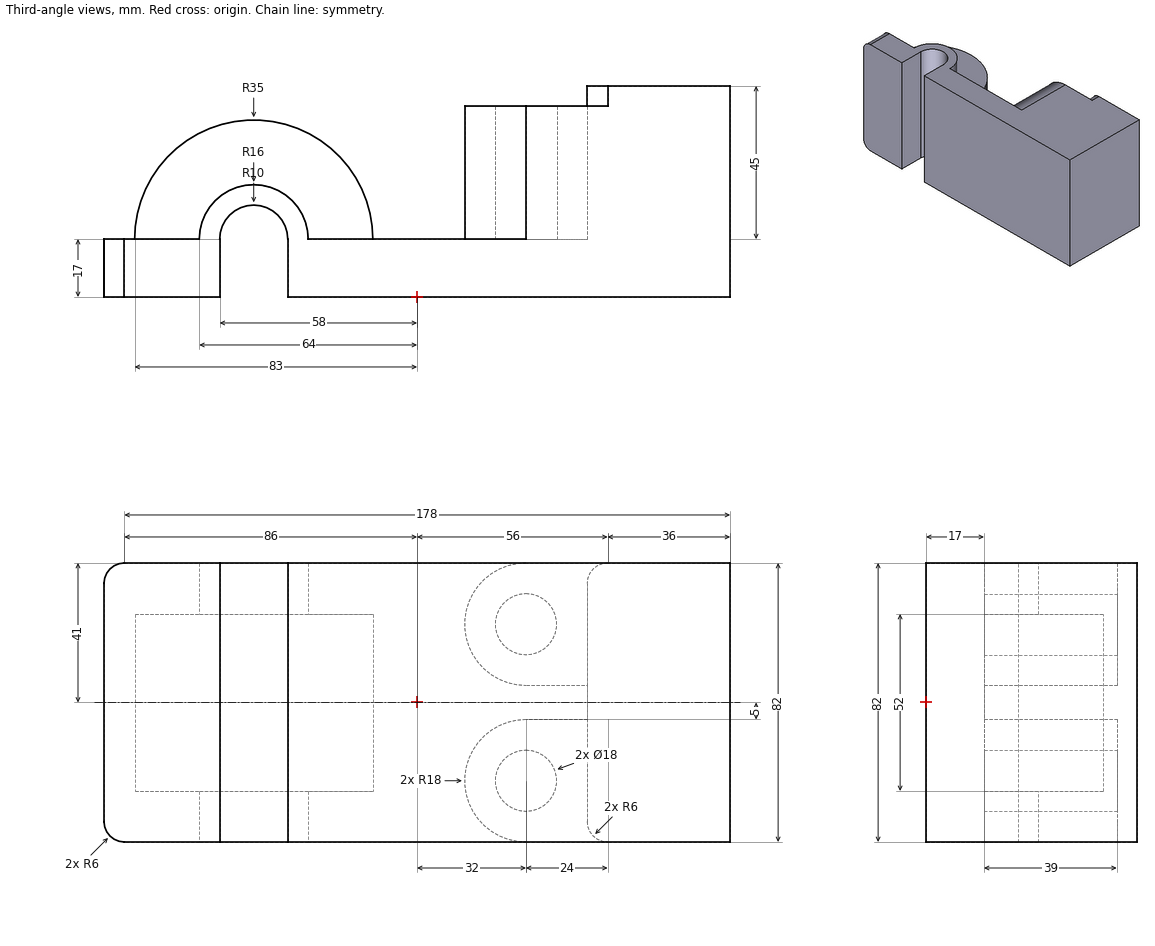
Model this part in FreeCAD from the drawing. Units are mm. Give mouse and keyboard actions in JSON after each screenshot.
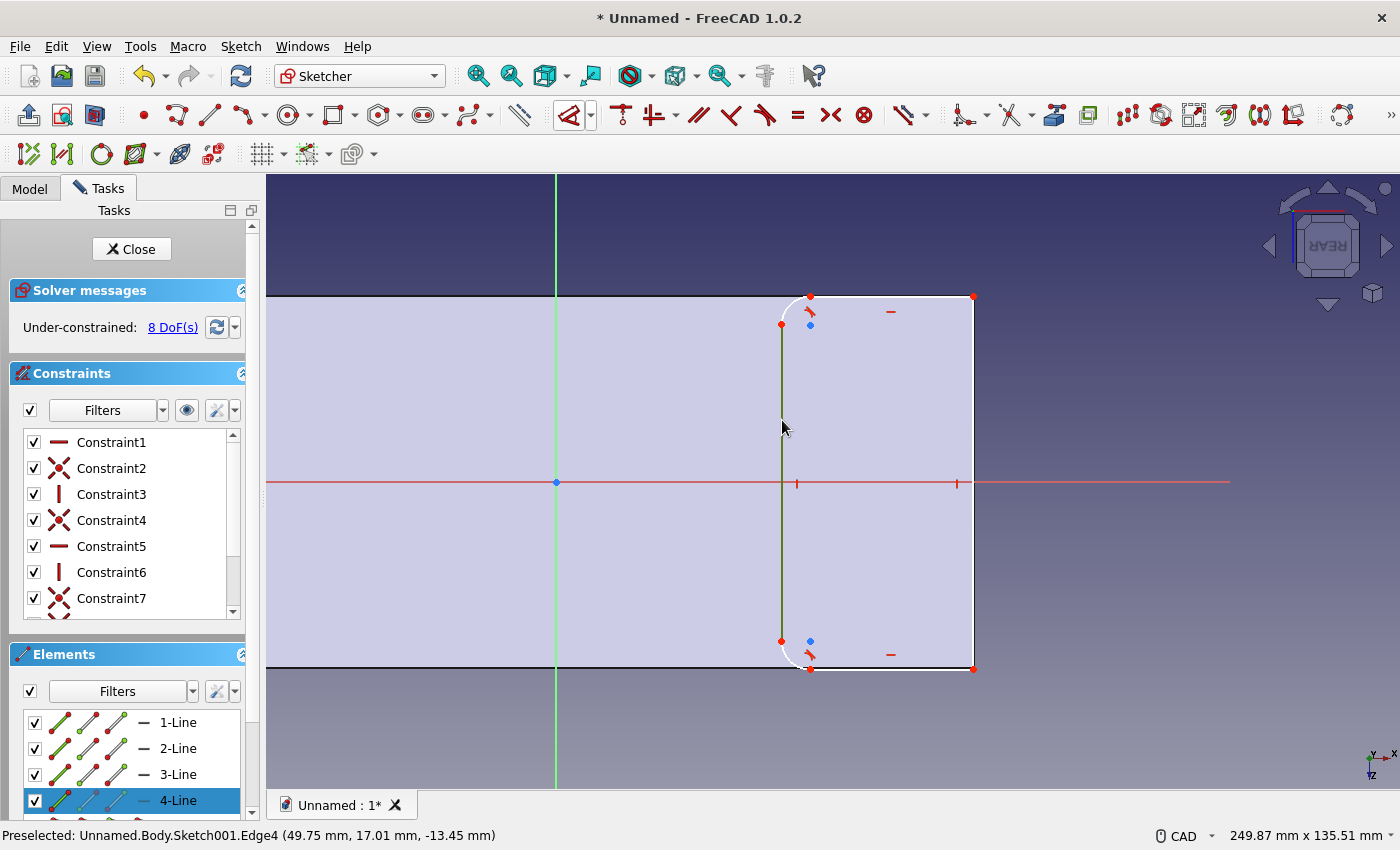
{"action": "left_click", "coordinate": [797, 300]}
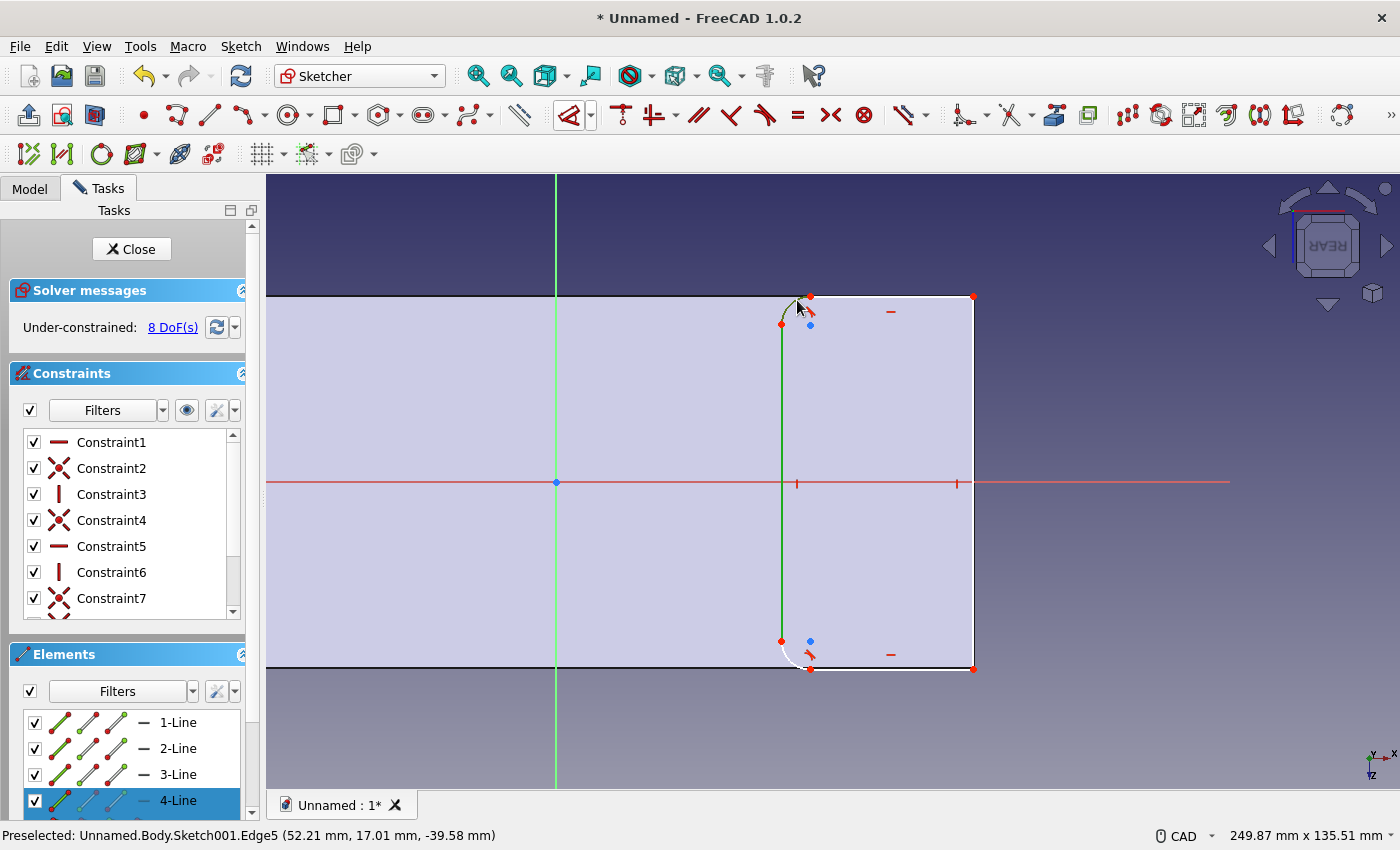
{"action": "left_click", "coordinate": [765, 116]}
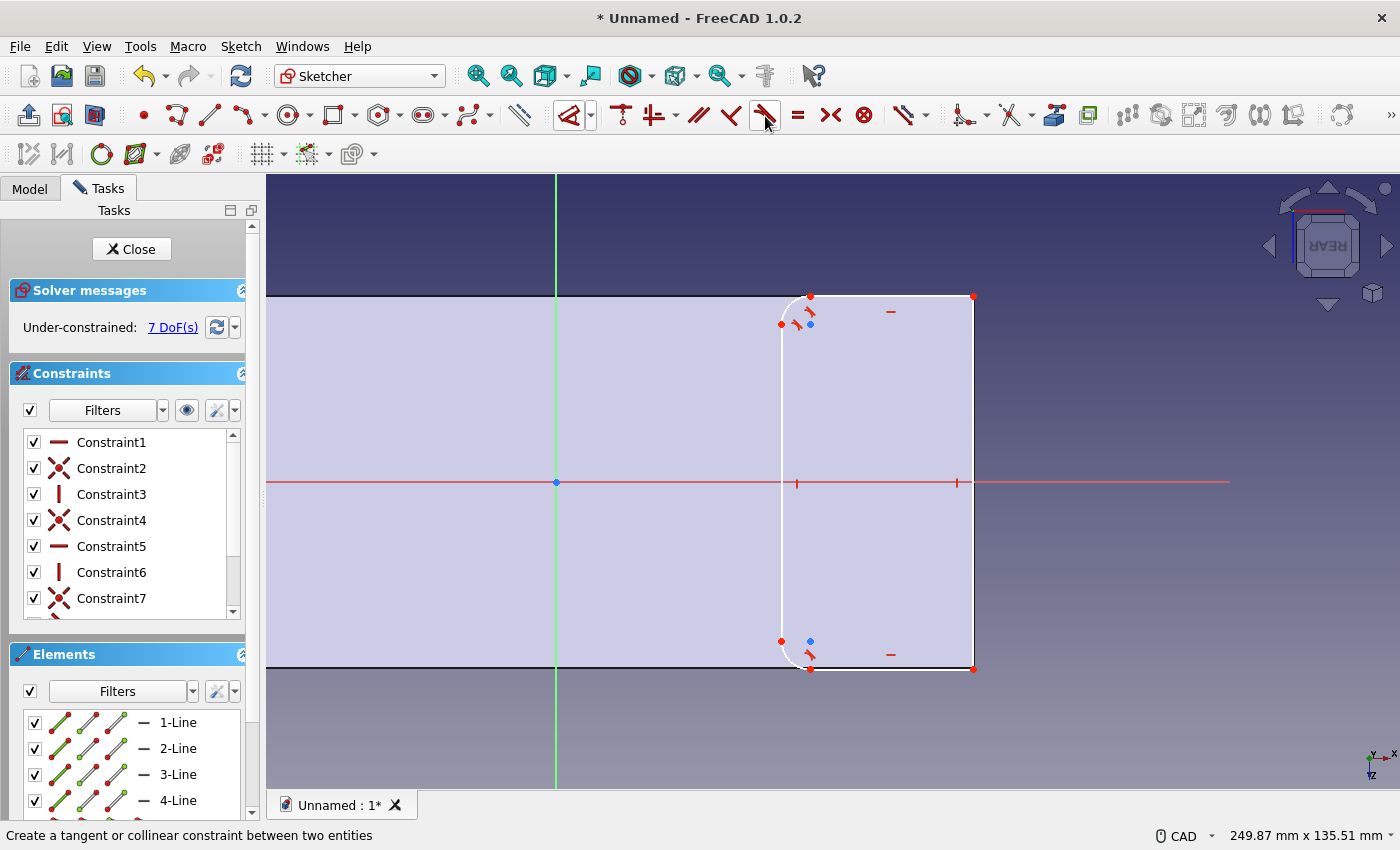
{"action": "left_click", "coordinate": [782, 420]}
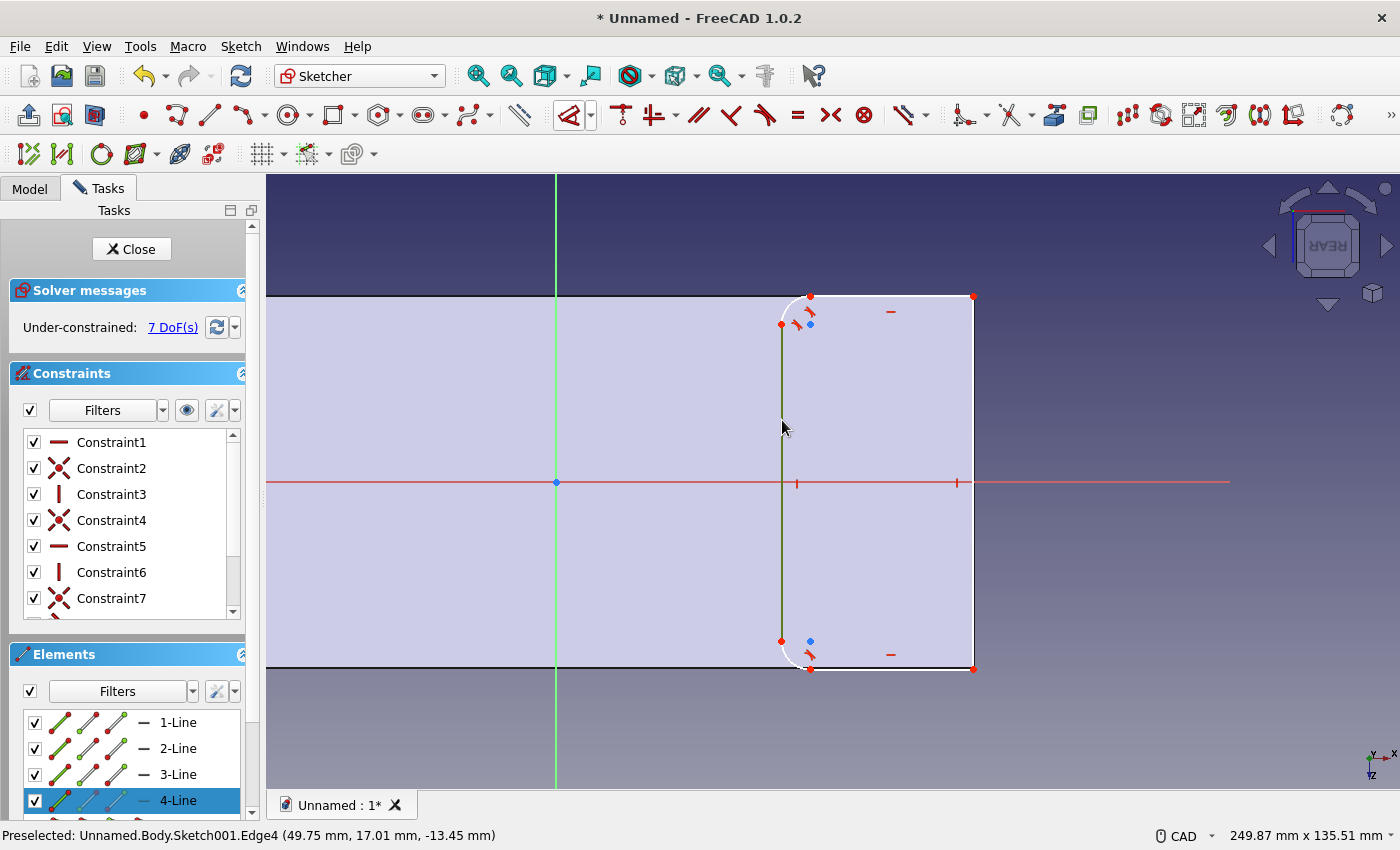
{"action": "left_click", "coordinate": [785, 654]}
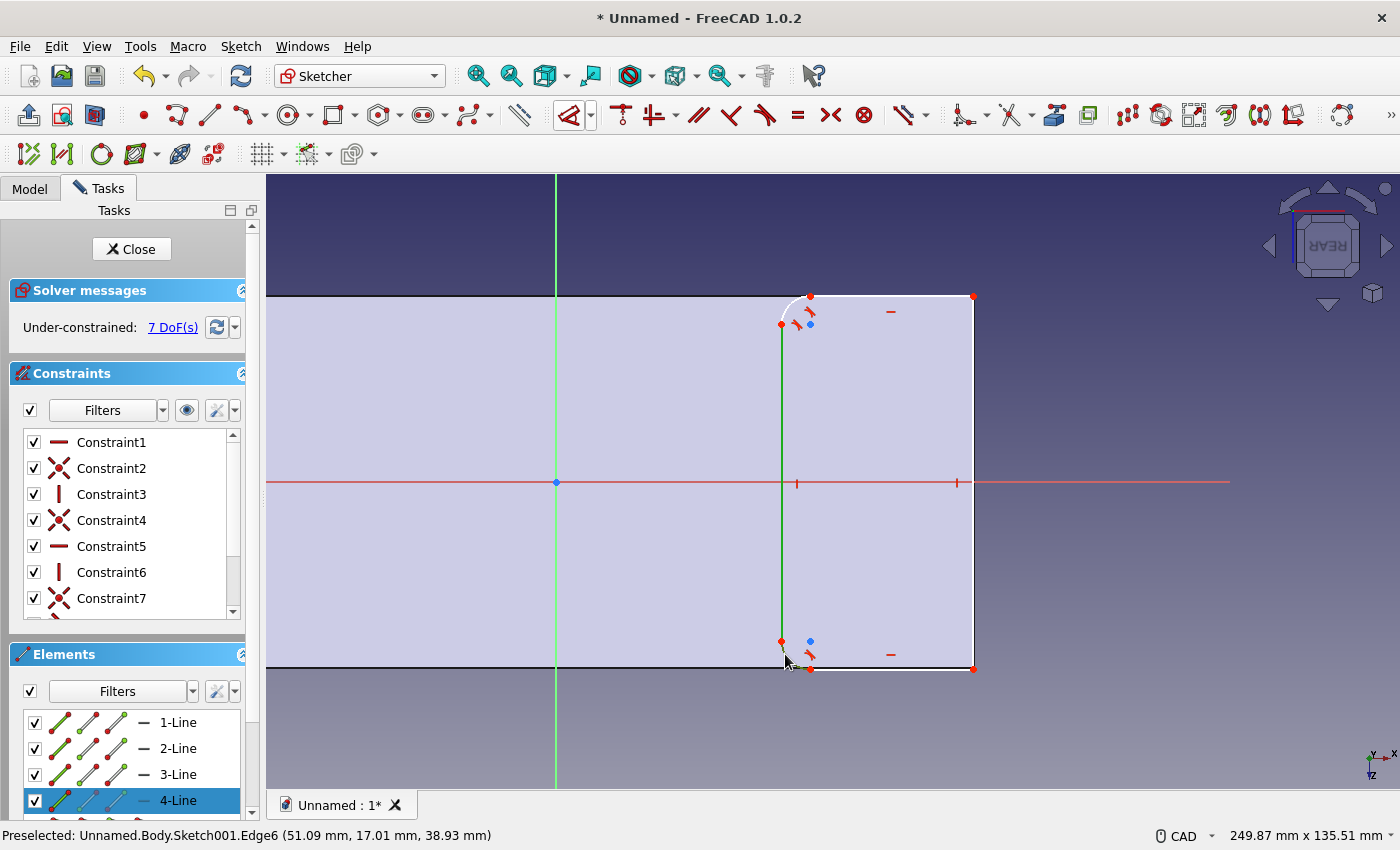
{"action": "left_click", "coordinate": [765, 116]}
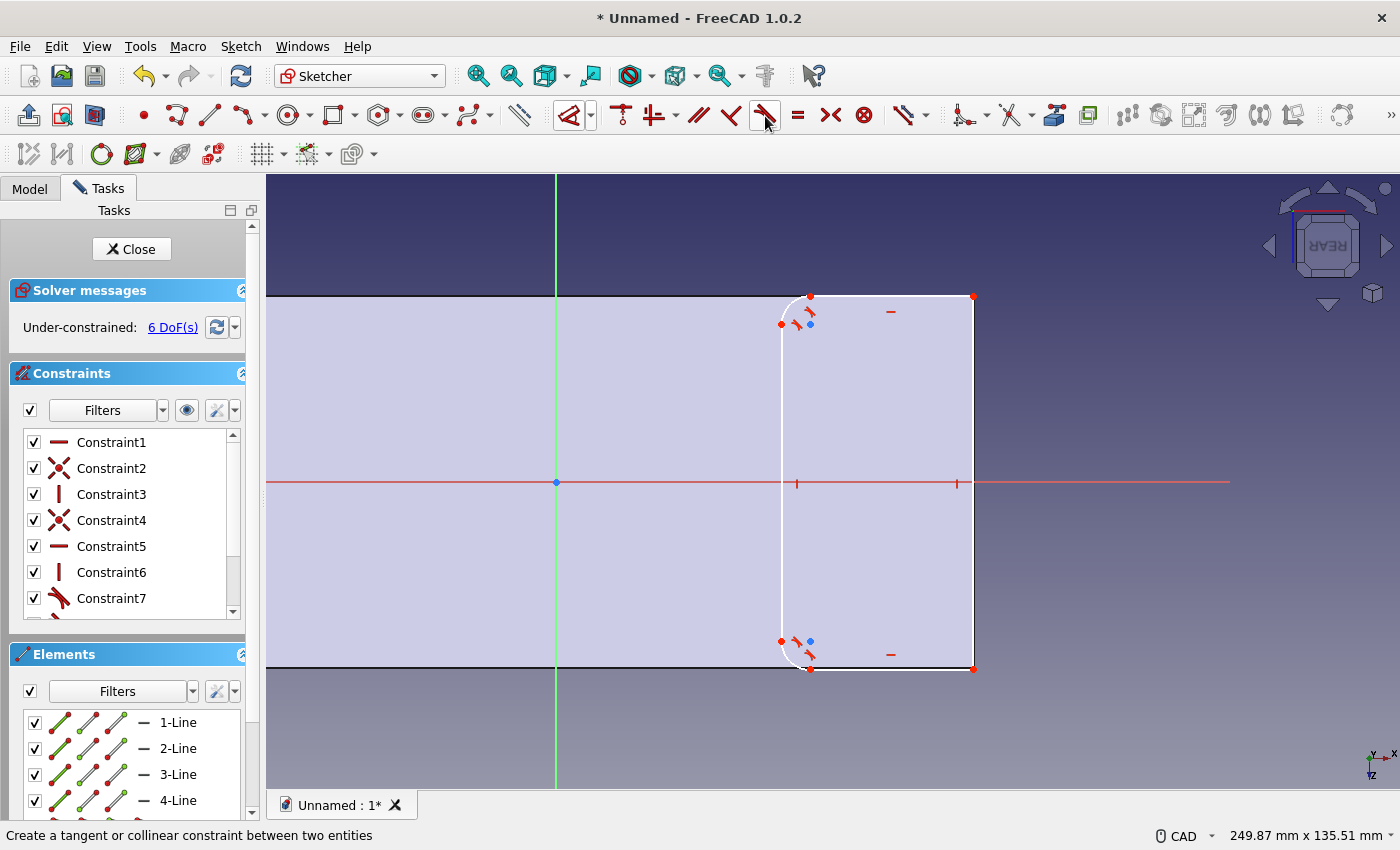
{"action": "left_click", "coordinate": [797, 299]}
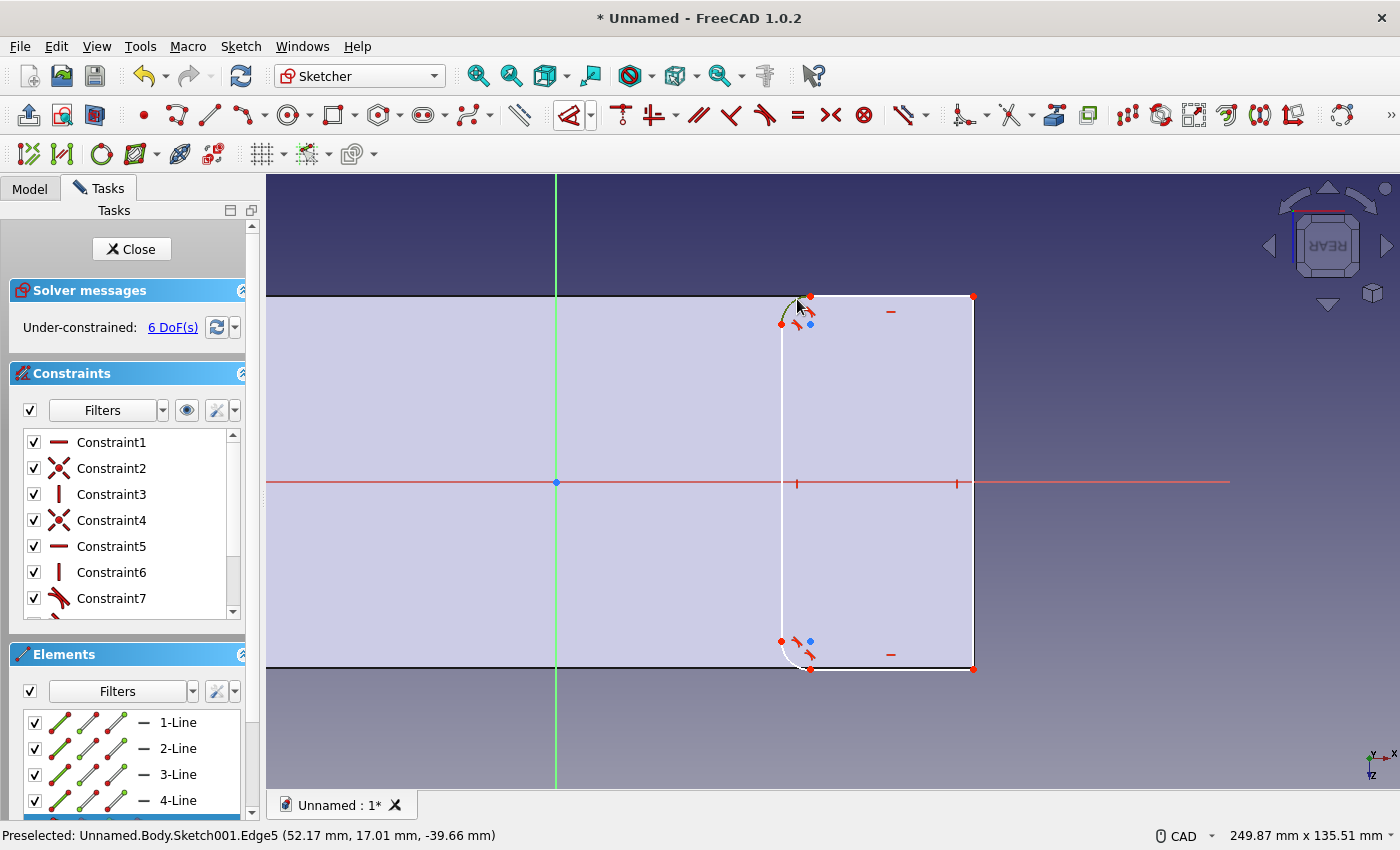
{"action": "left_click", "coordinate": [785, 654]}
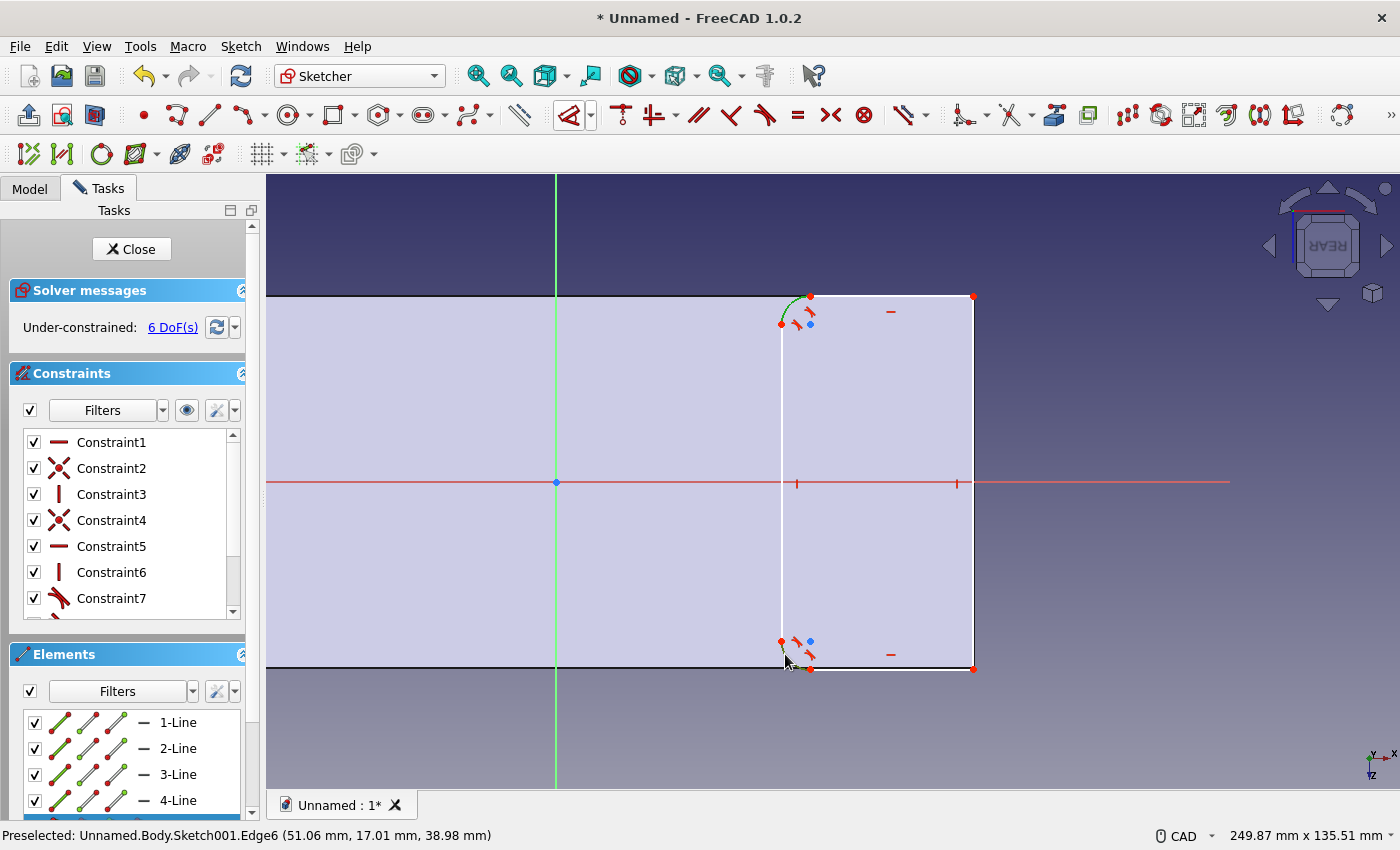
{"action": "left_click", "coordinate": [798, 116]}